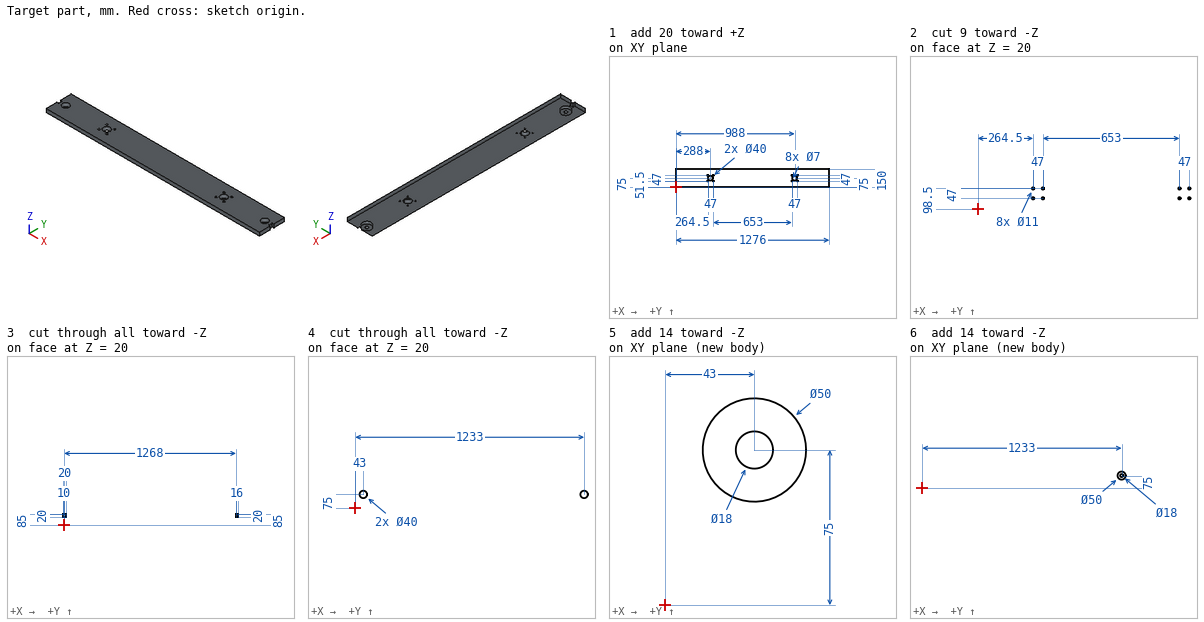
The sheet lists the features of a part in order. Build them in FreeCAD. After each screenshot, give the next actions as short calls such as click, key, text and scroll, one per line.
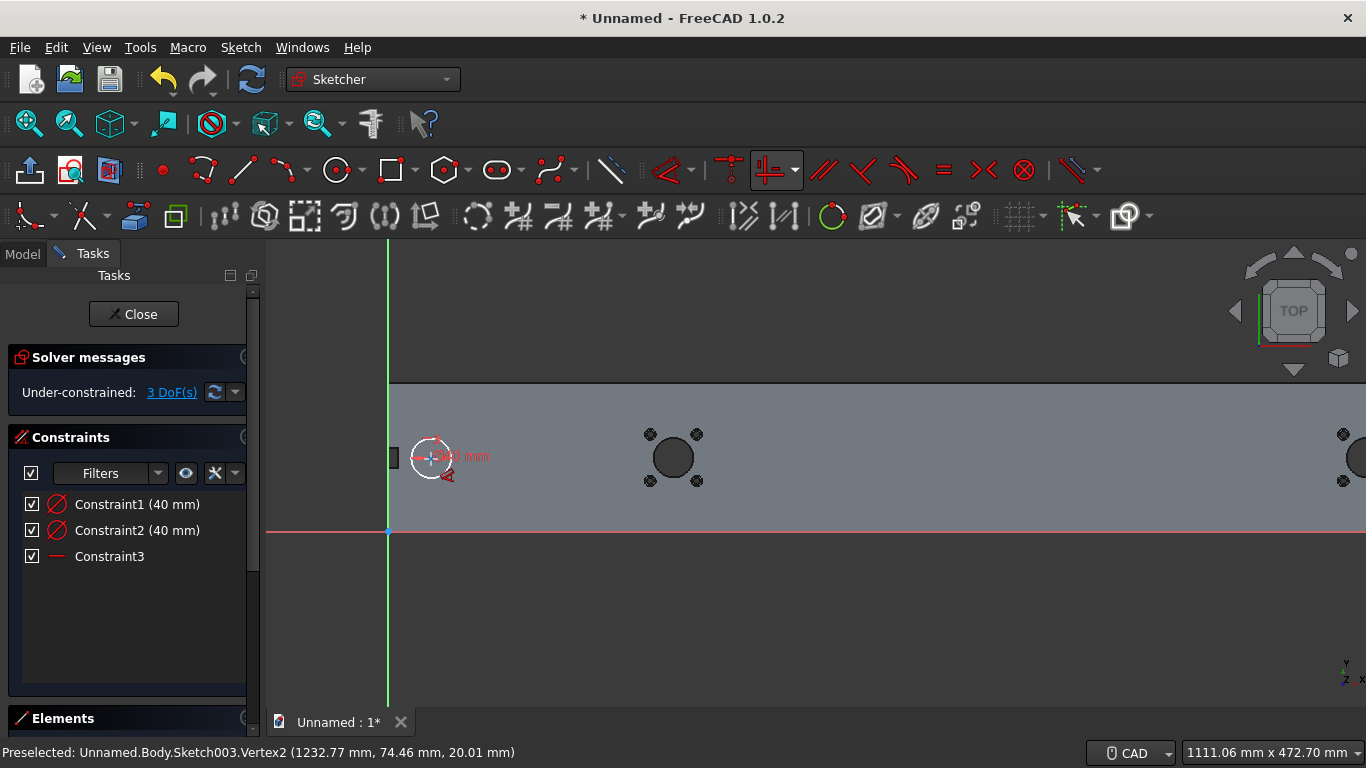
click(431, 458)
click(410, 566)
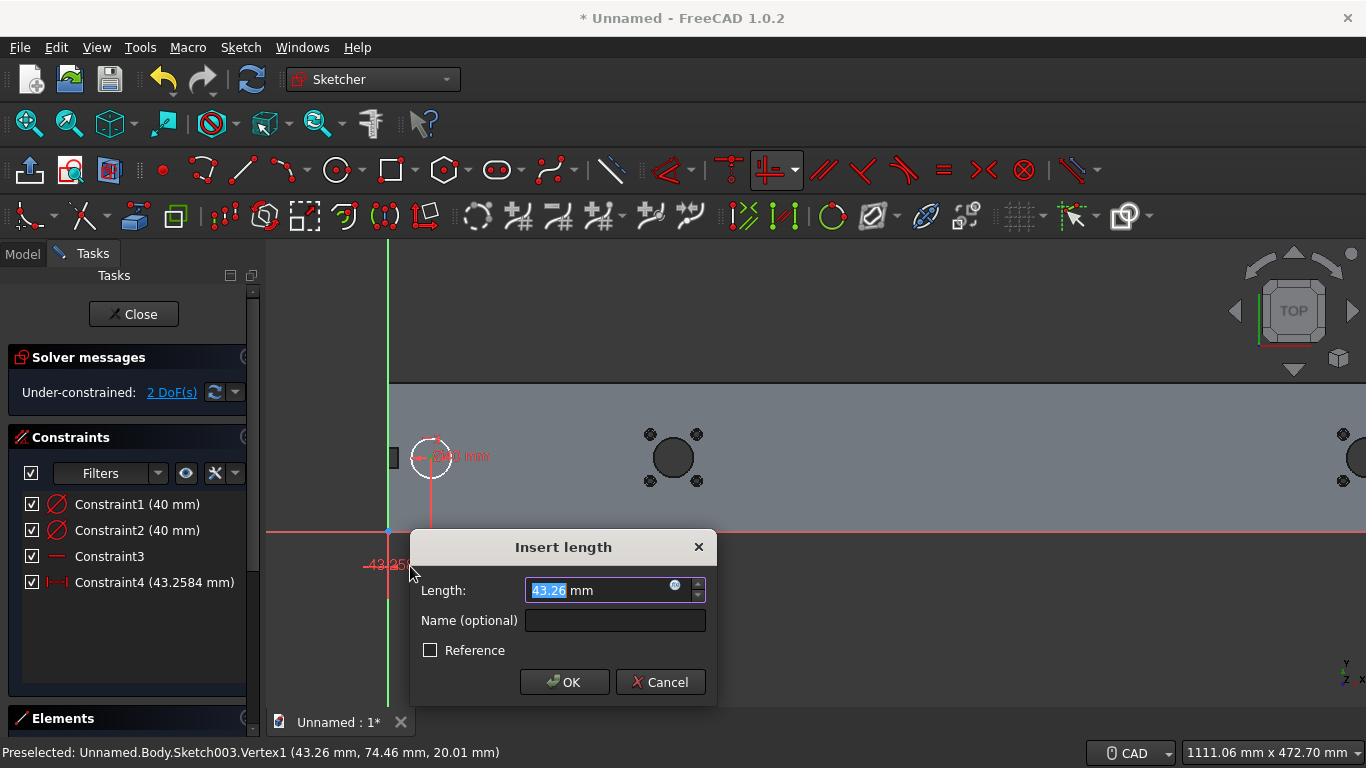
text(43)
key(Return)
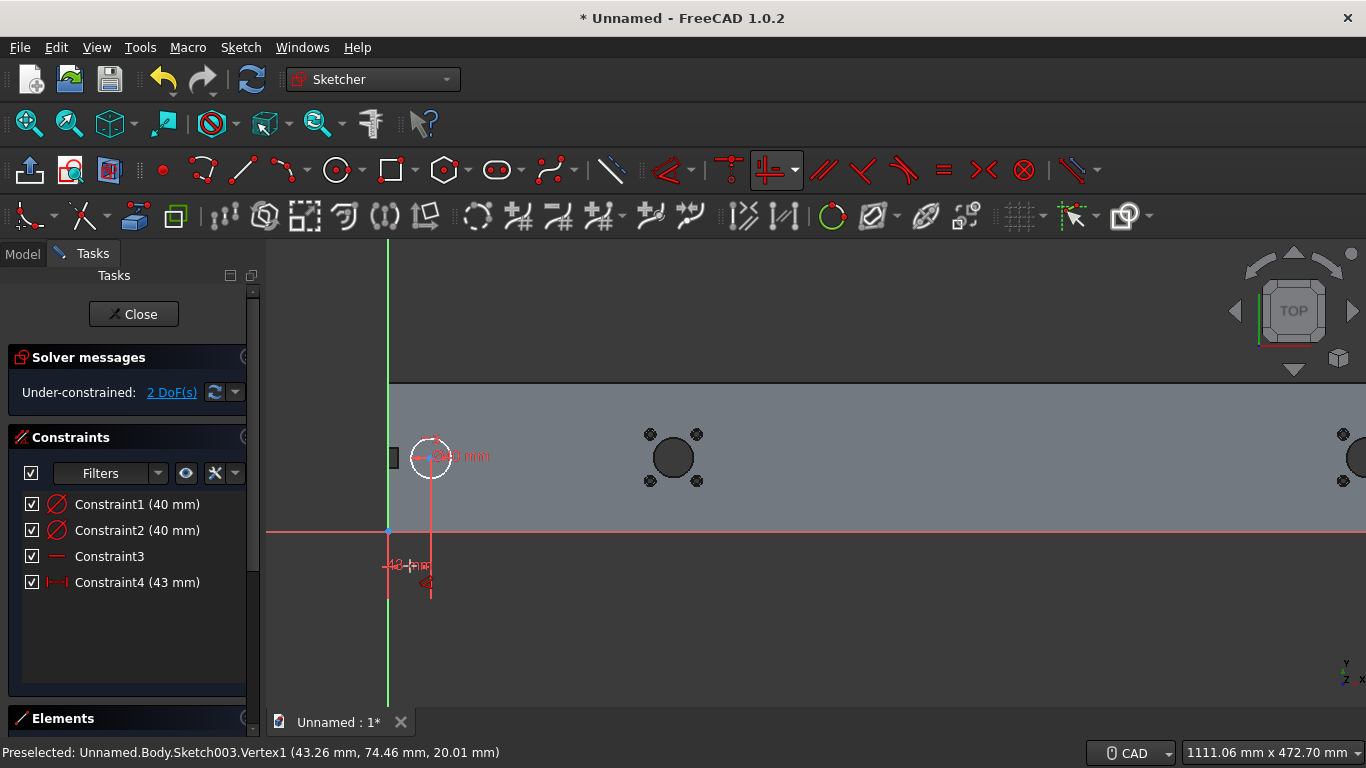
click(431, 458)
click(354, 495)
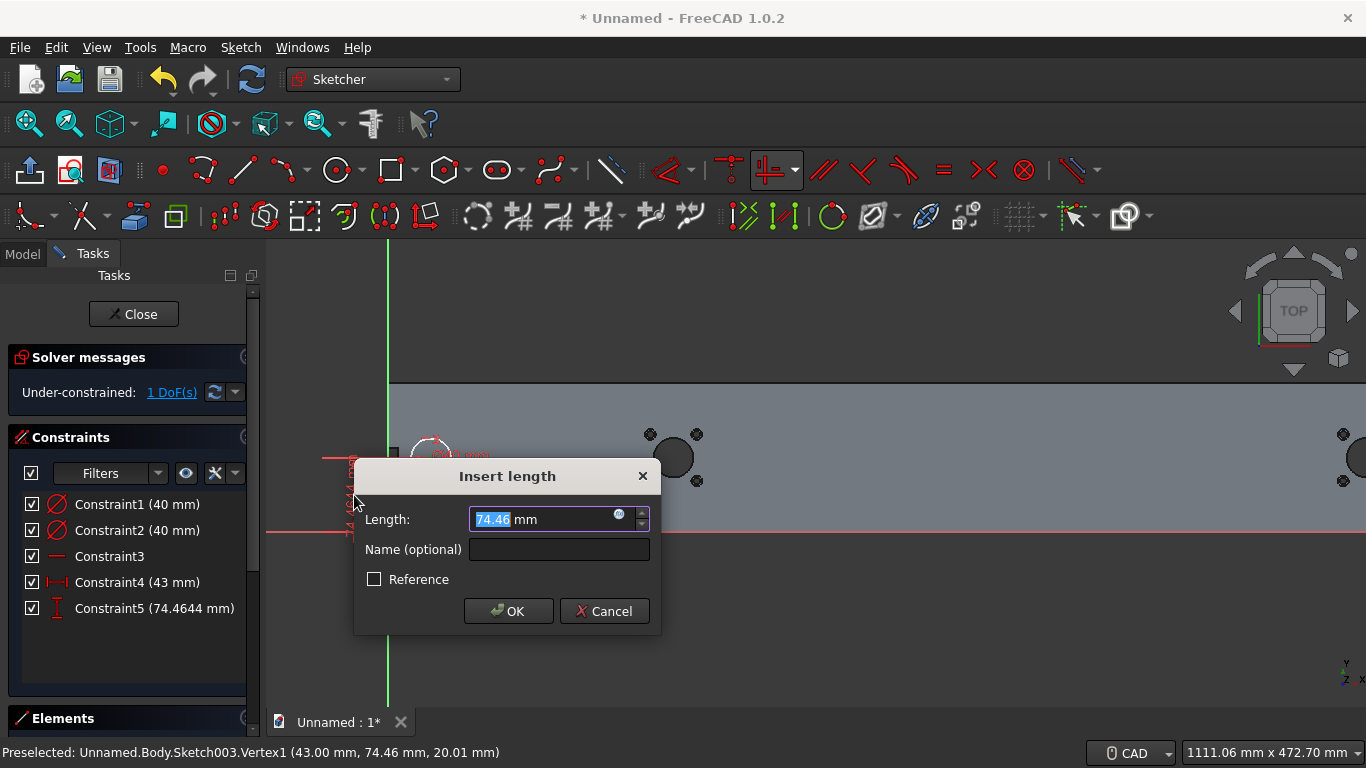
text(75)
key(Return)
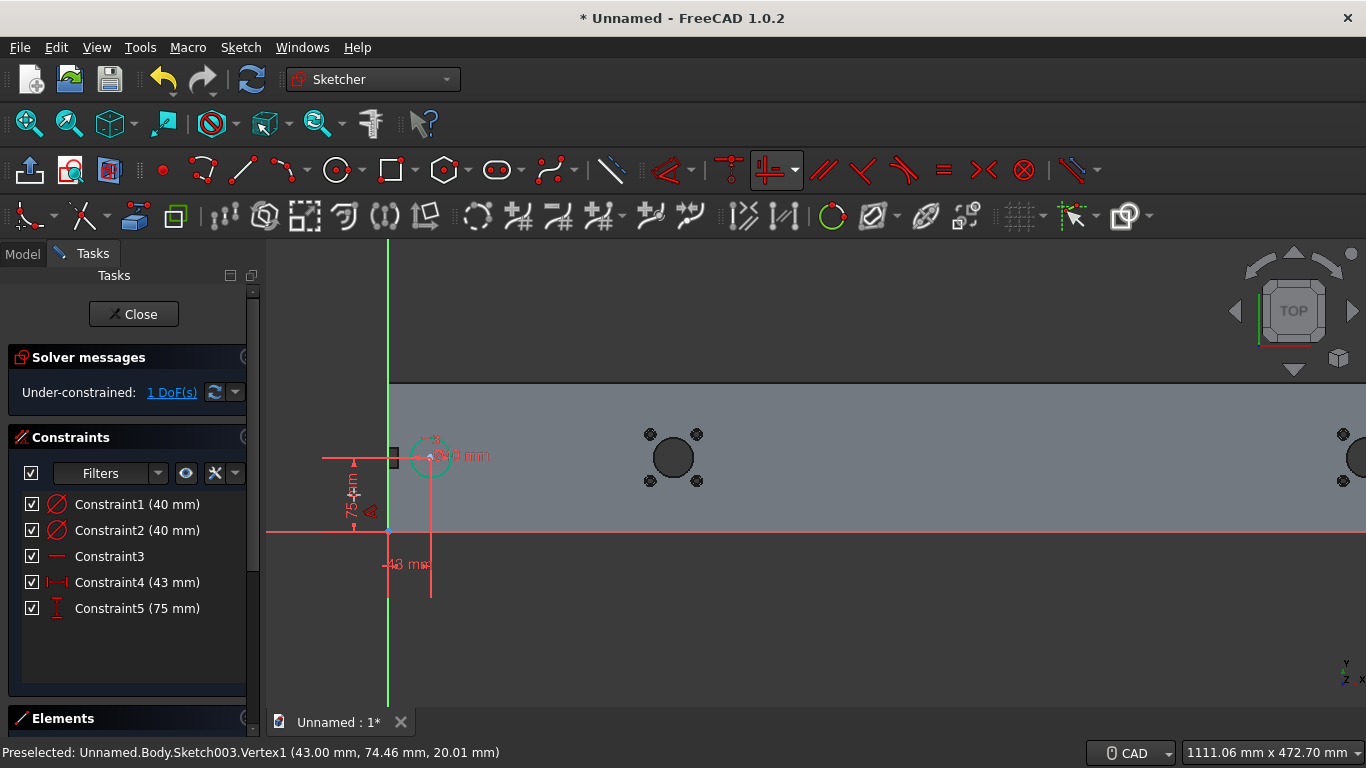
scroll(430, 458, down, 3)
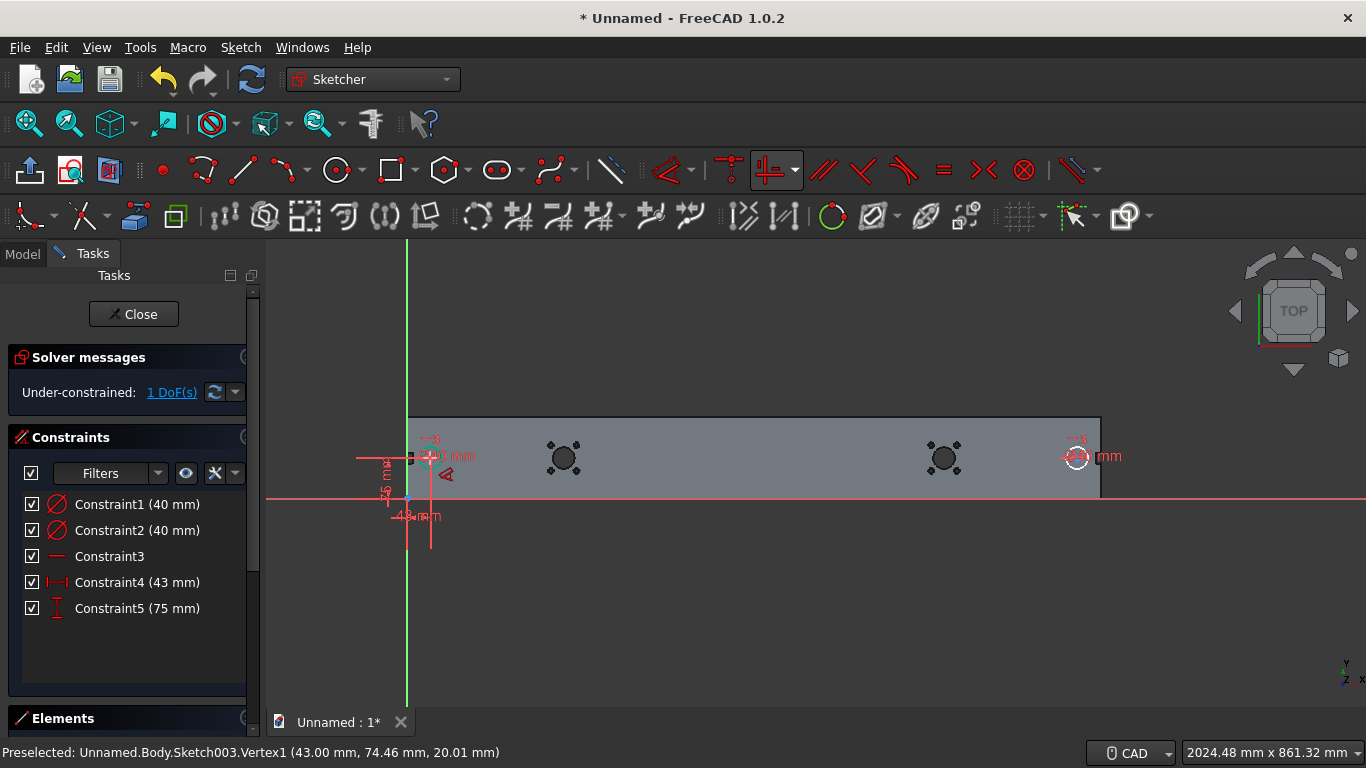
click(1077, 458)
click(742, 533)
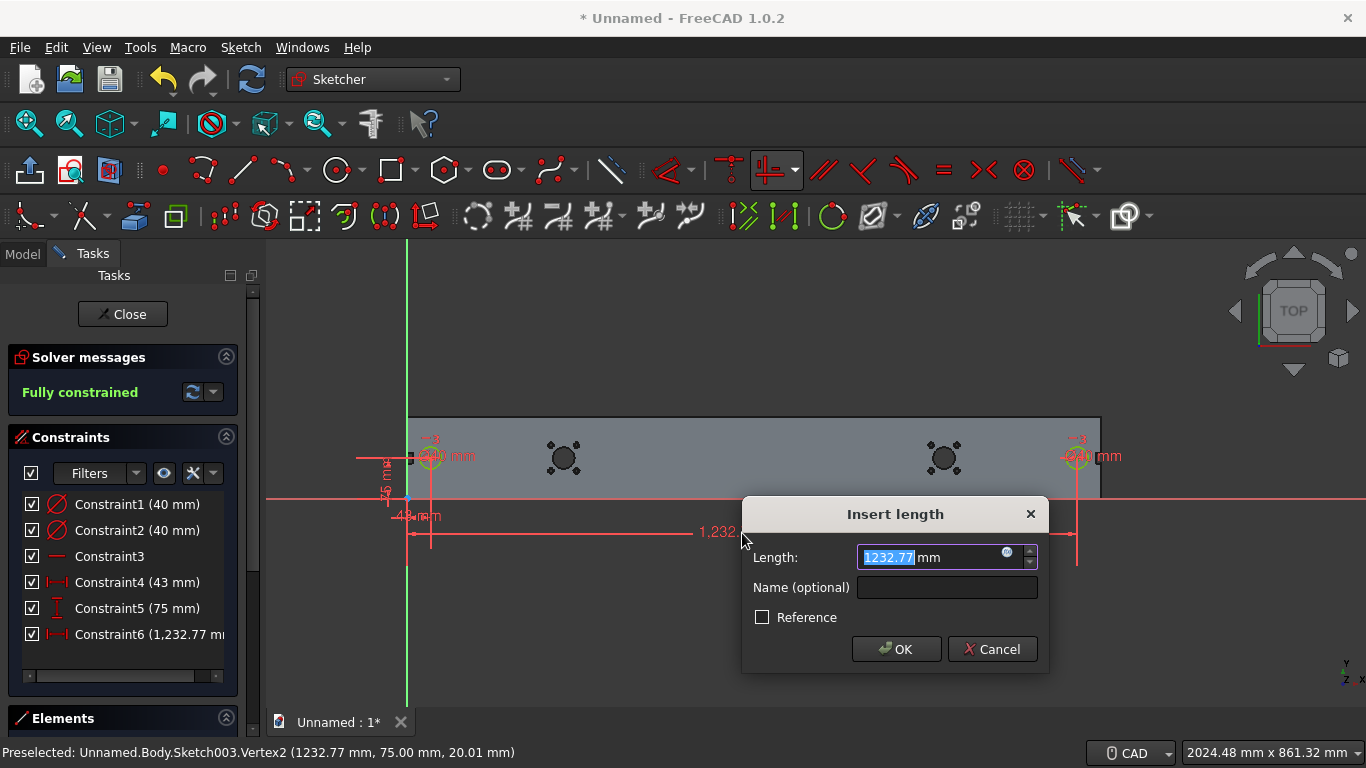
text(1233)
key(Return)
key(Escape)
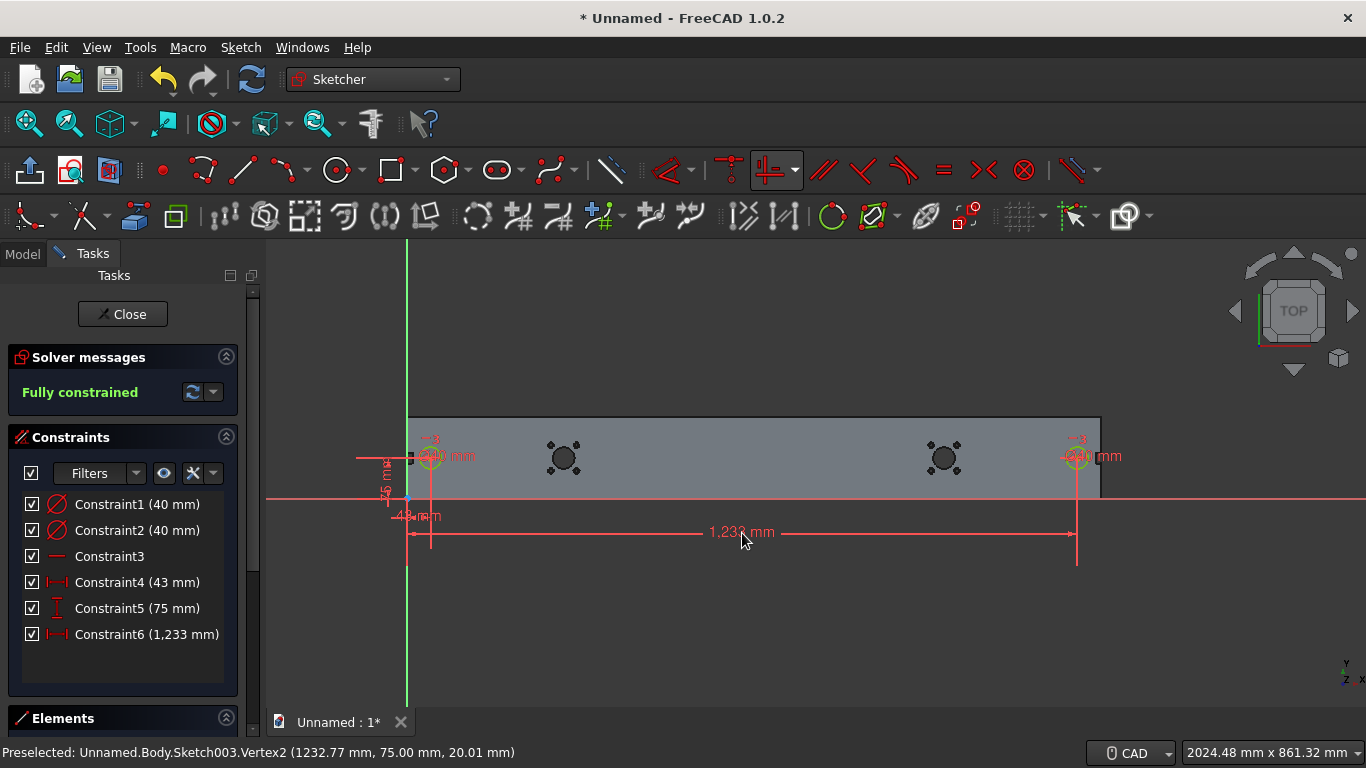
click(123, 314)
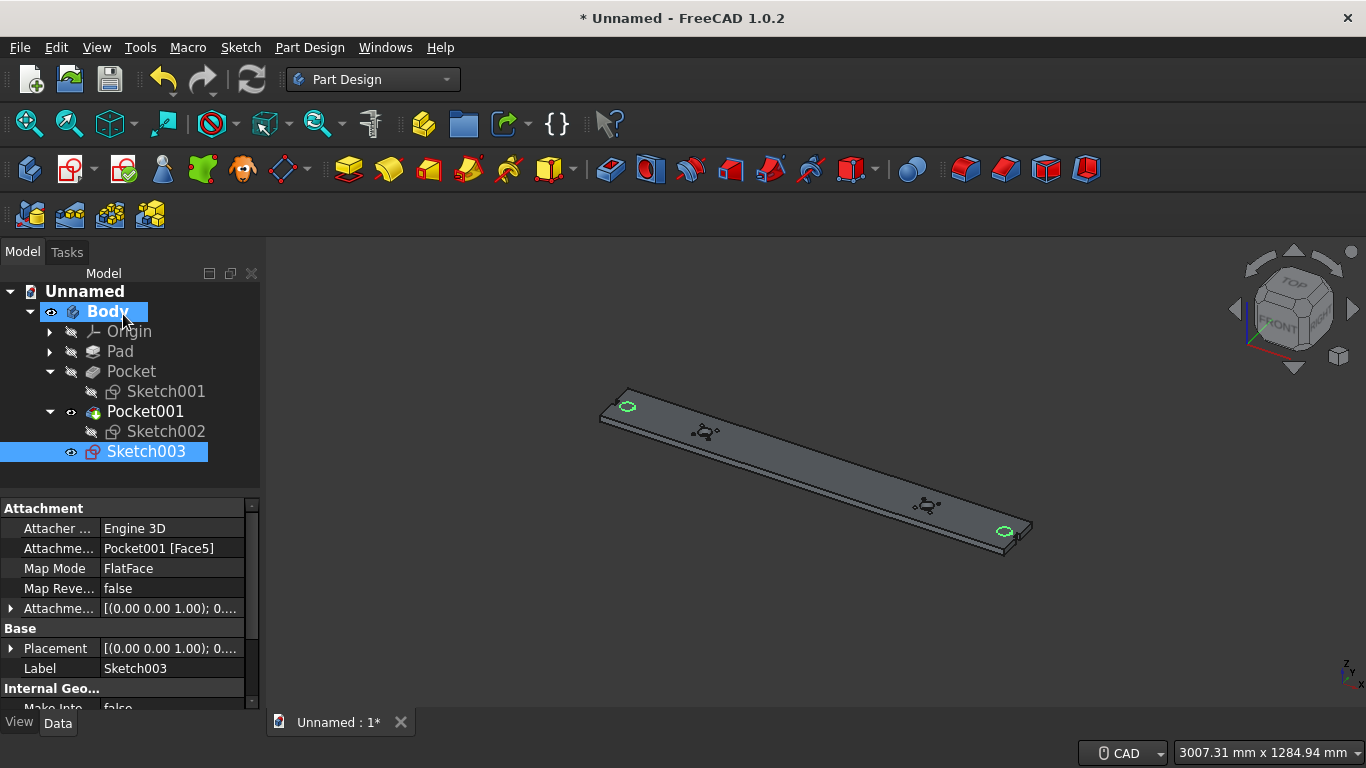
click(612, 170)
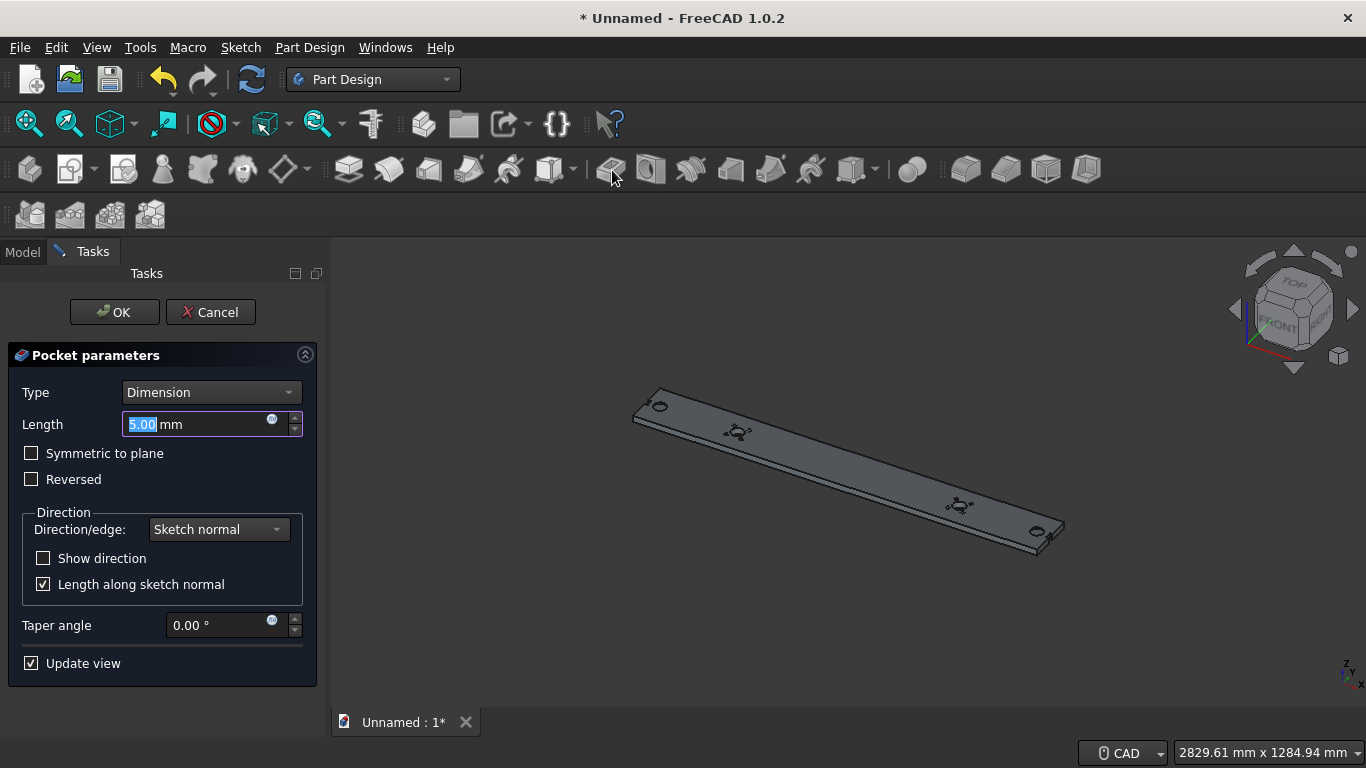
click(212, 392)